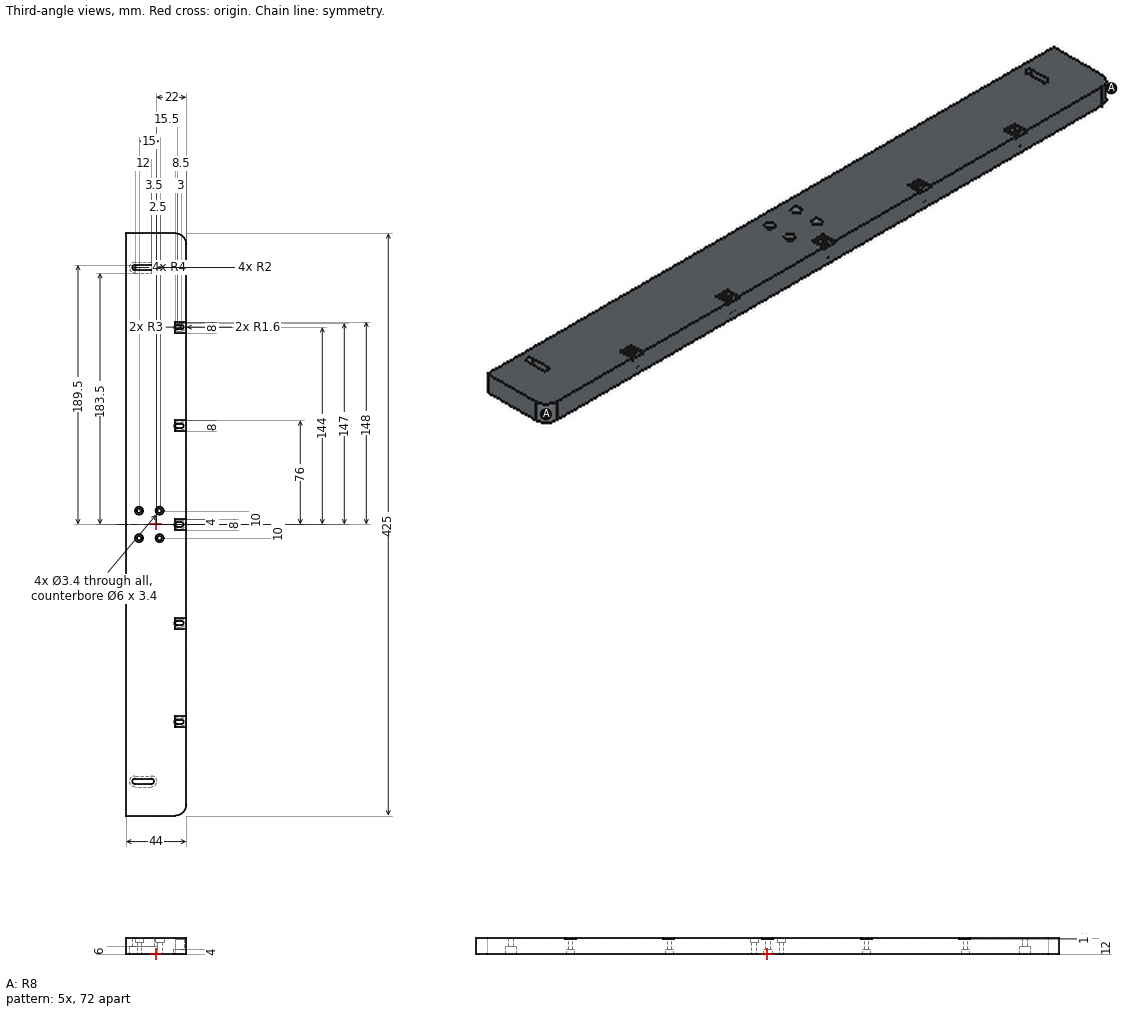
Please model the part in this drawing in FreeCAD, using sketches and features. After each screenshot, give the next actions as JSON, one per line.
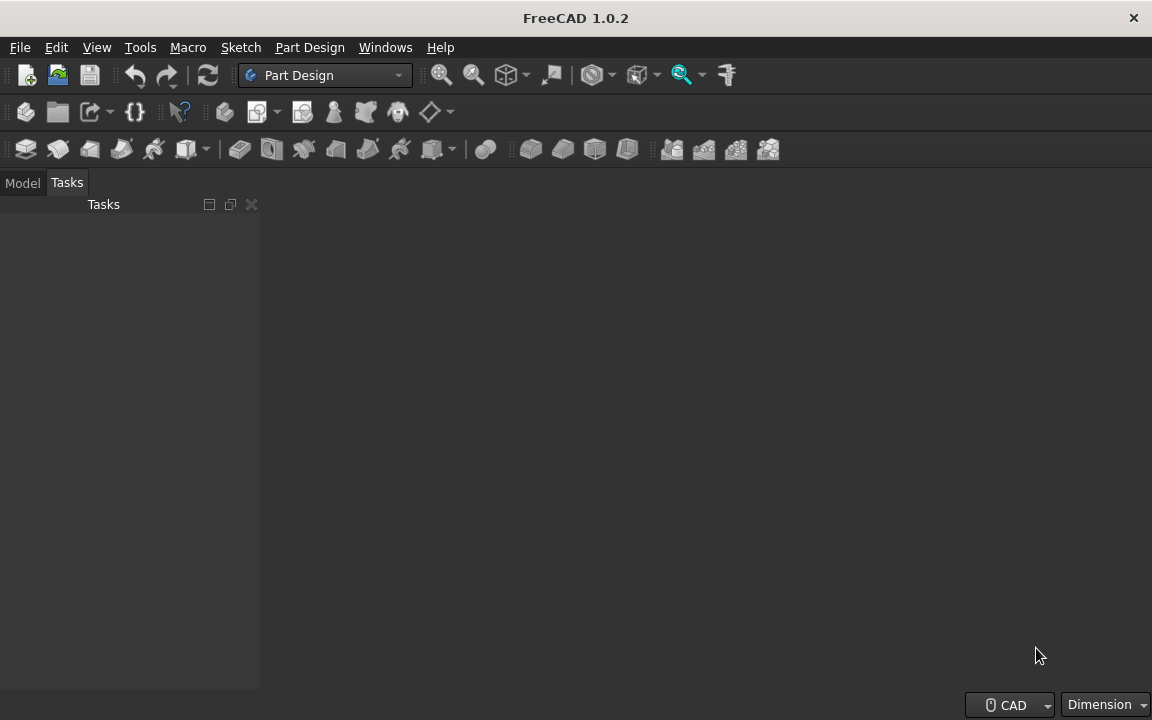
{"action": "key", "text": "ctrl+n"}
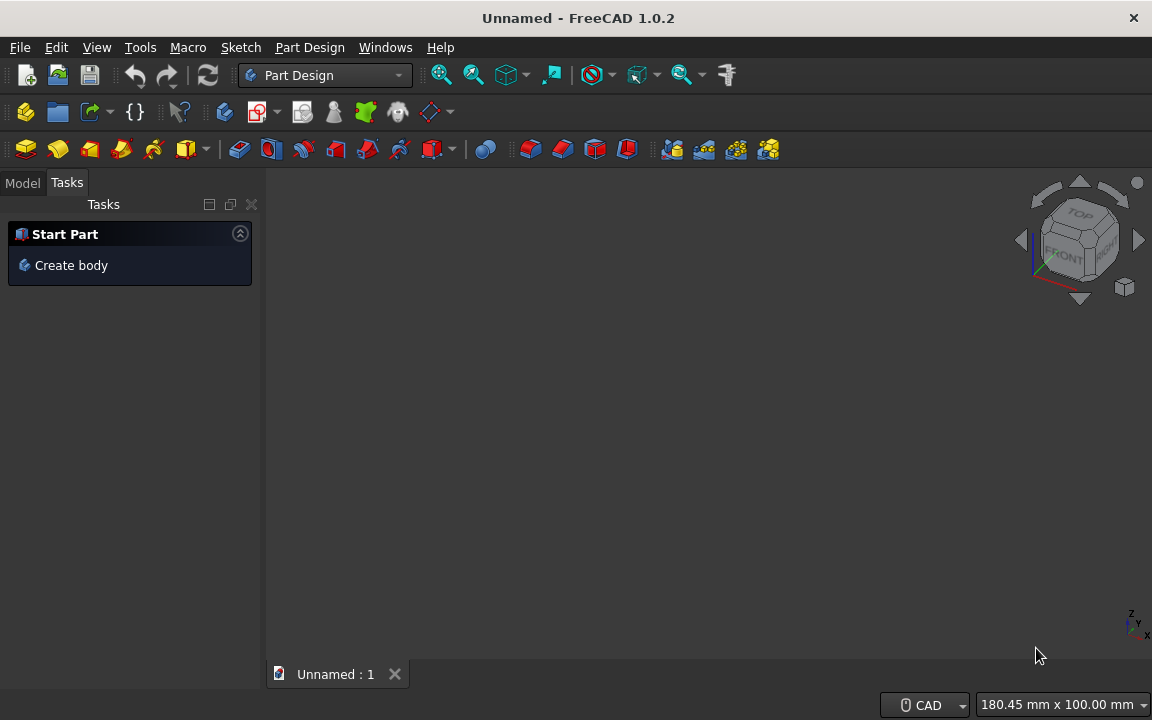
{"action": "left_click", "coordinate": [258, 112]}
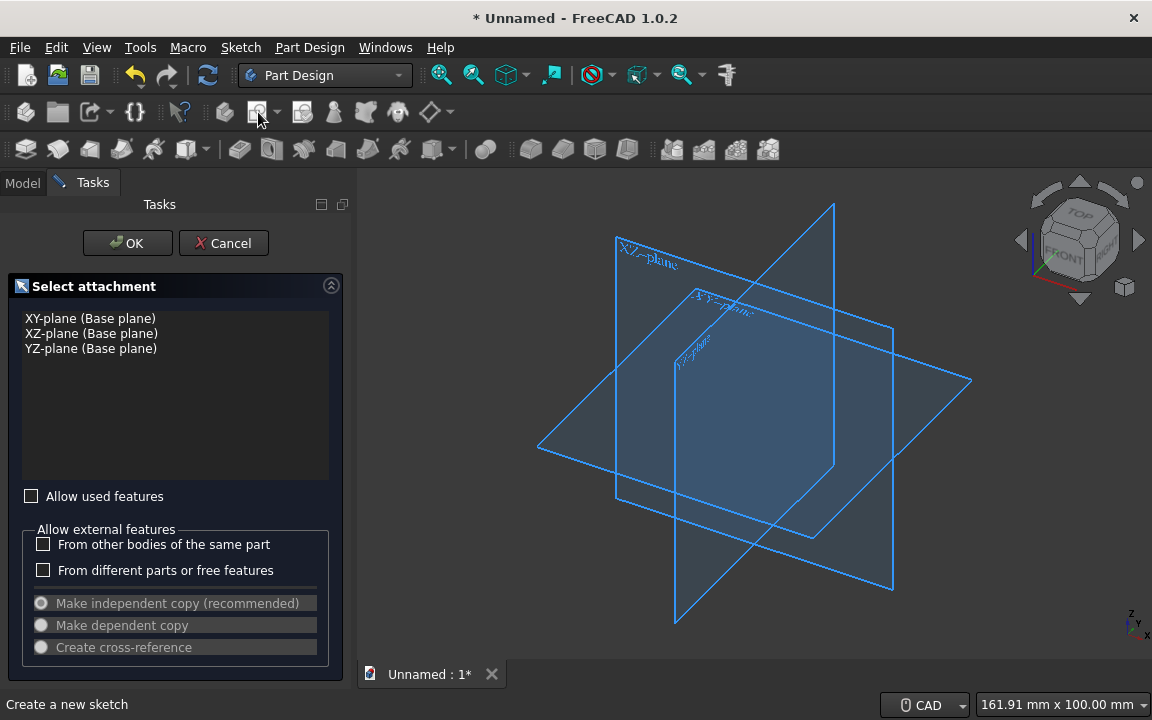
{"action": "left_click", "coordinate": [82, 318]}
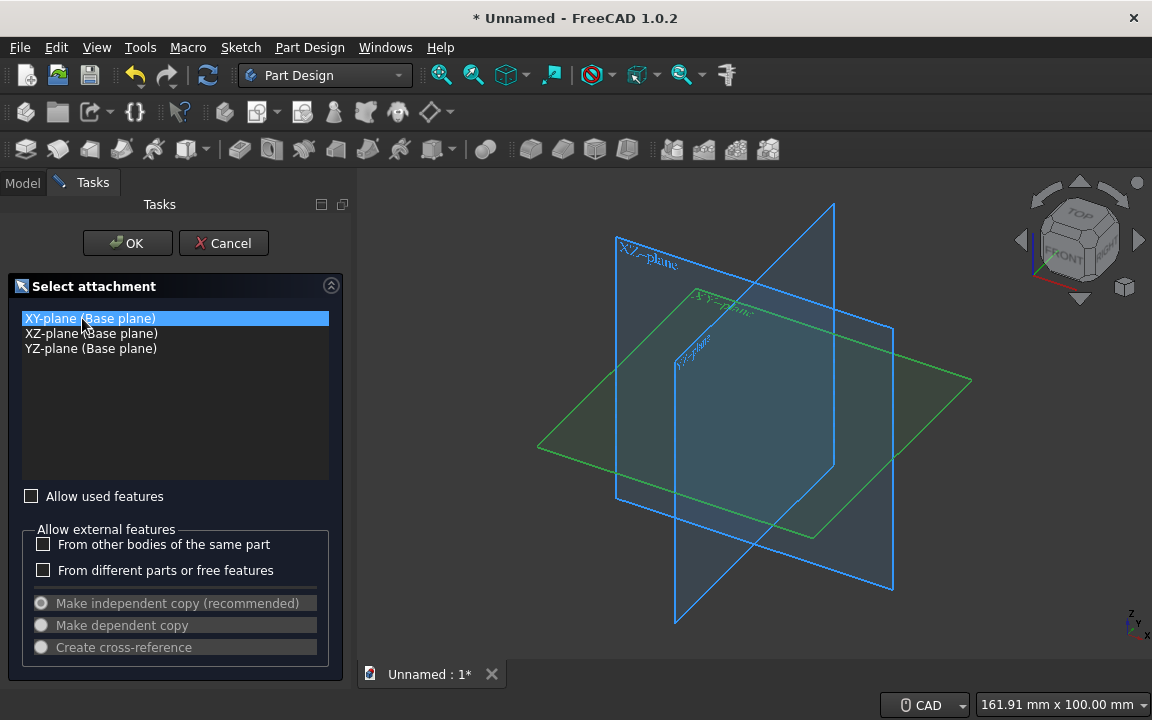
{"action": "left_click", "coordinate": [128, 243]}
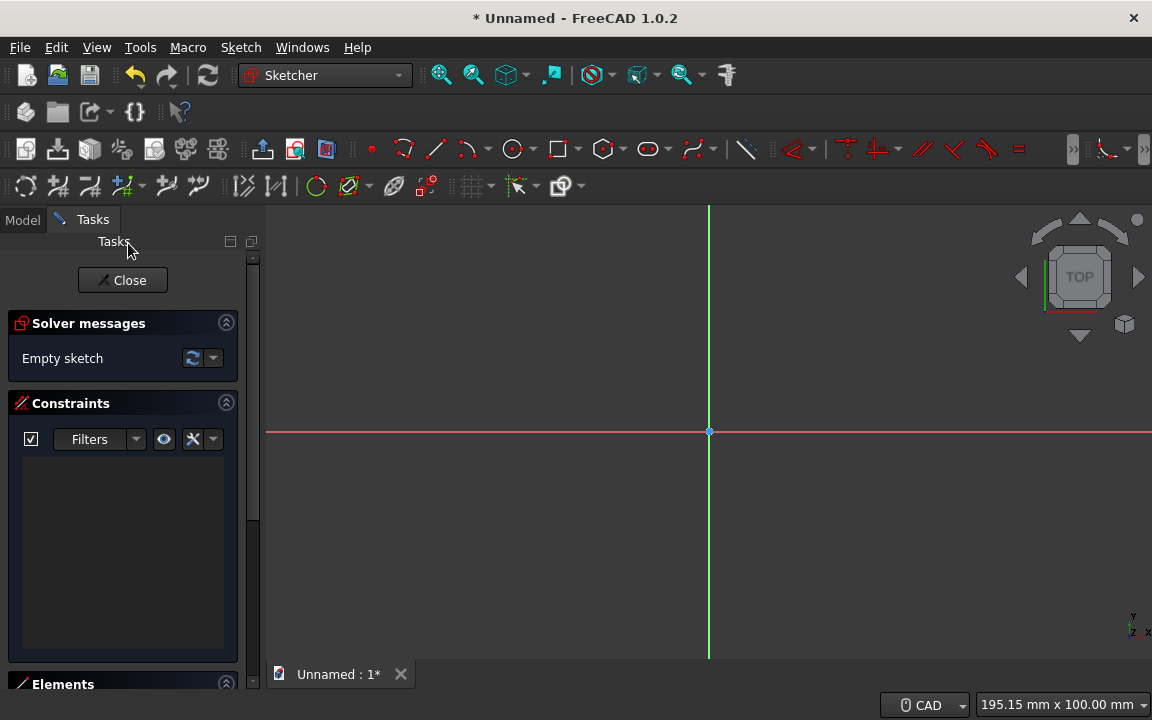
{"action": "scroll", "coordinate": [630, 432], "scroll_direction": "down", "scroll_amount": 10}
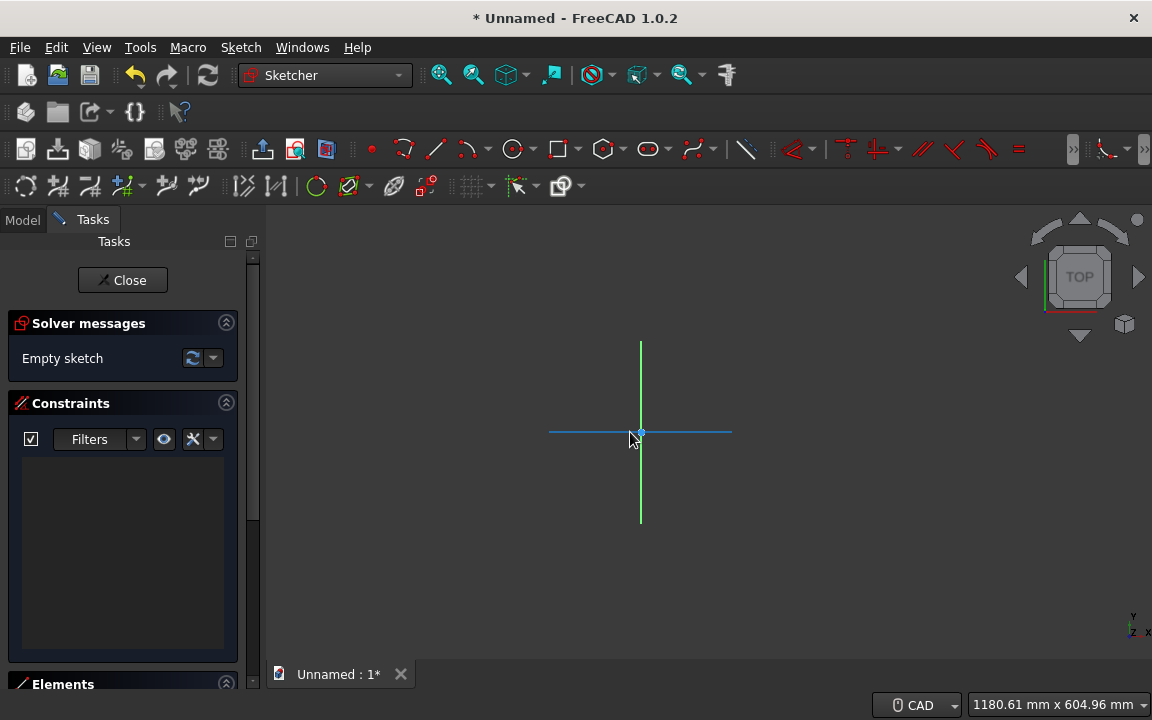
{"action": "key", "text": "g v"}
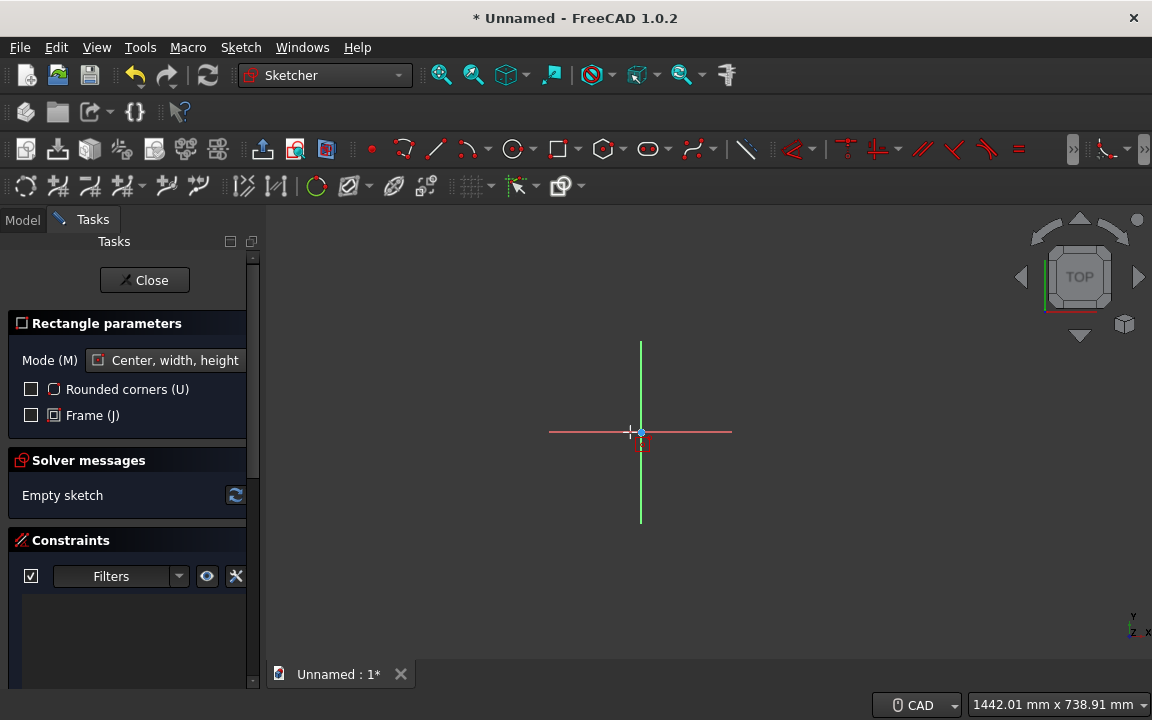
{"action": "left_click", "coordinate": [641, 432]}
{"action": "left_click", "coordinate": [655, 302]}
{"action": "key", "text": "Escape"}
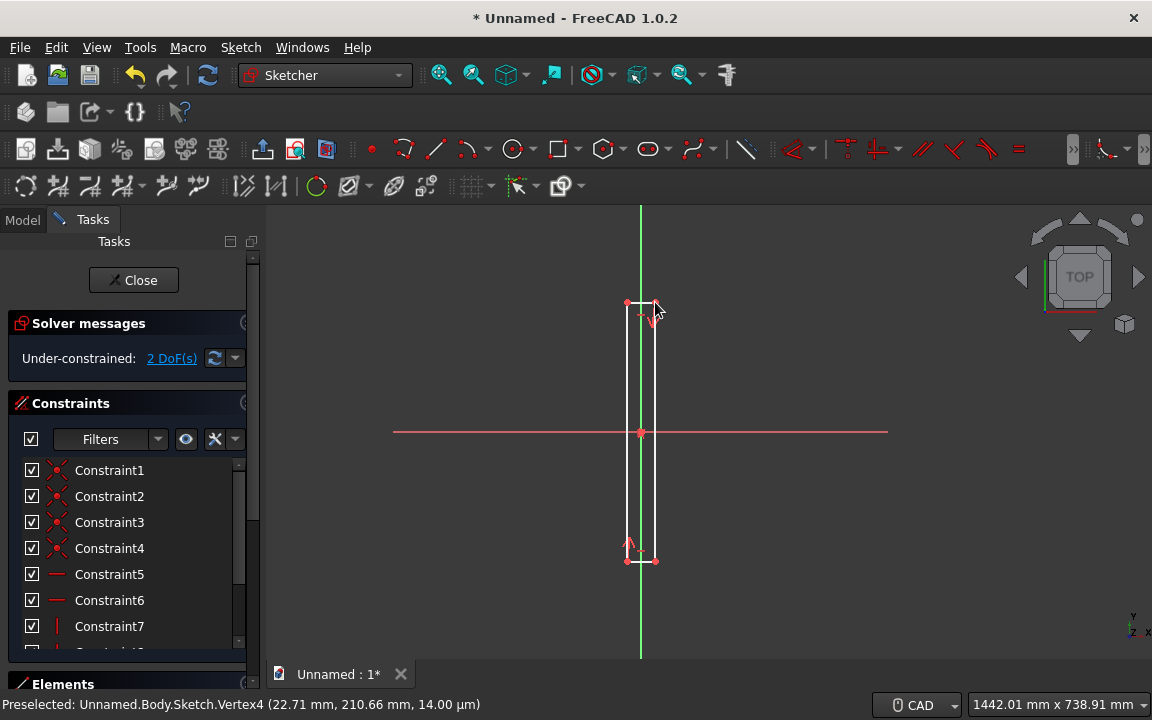
{"action": "scroll", "coordinate": [638, 562], "scroll_direction": "up", "scroll_amount": 2}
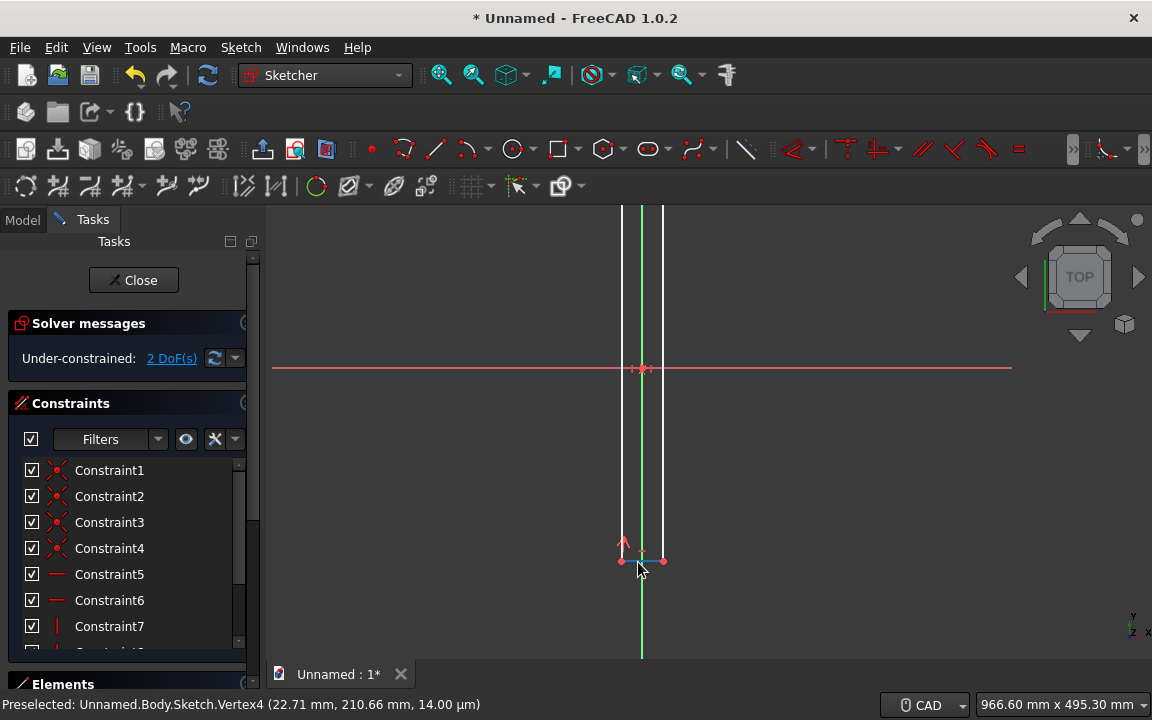
{"action": "left_click", "coordinate": [638, 561]}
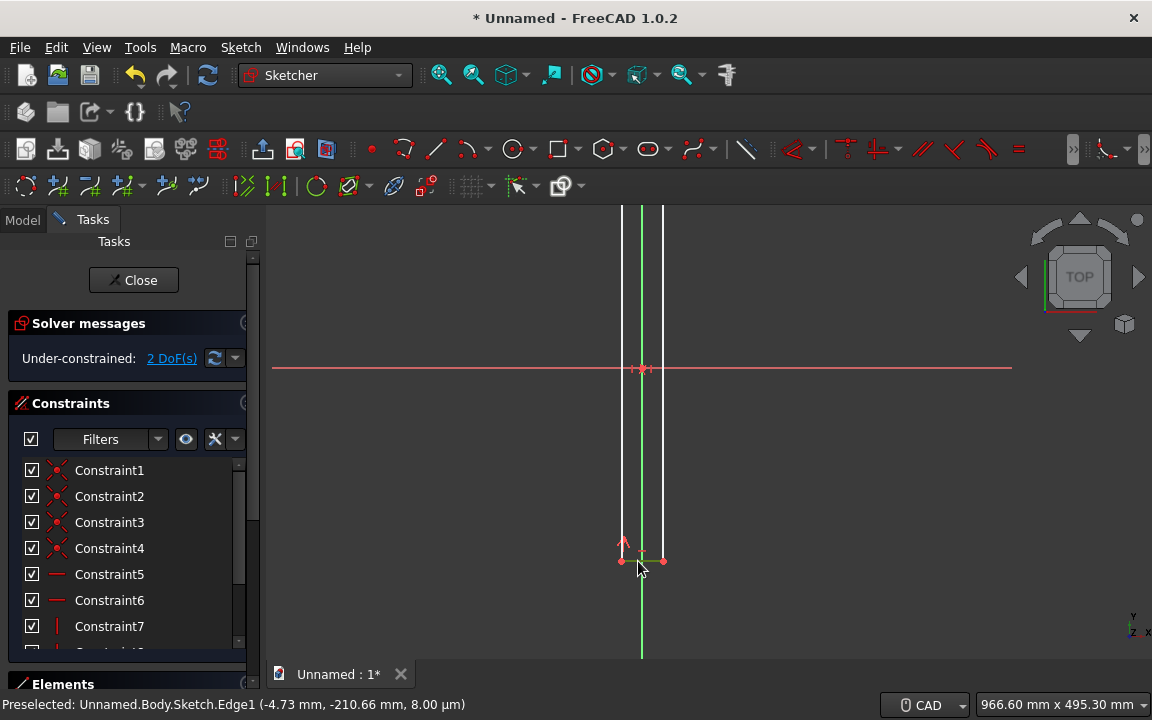
{"action": "key", "text": "l"}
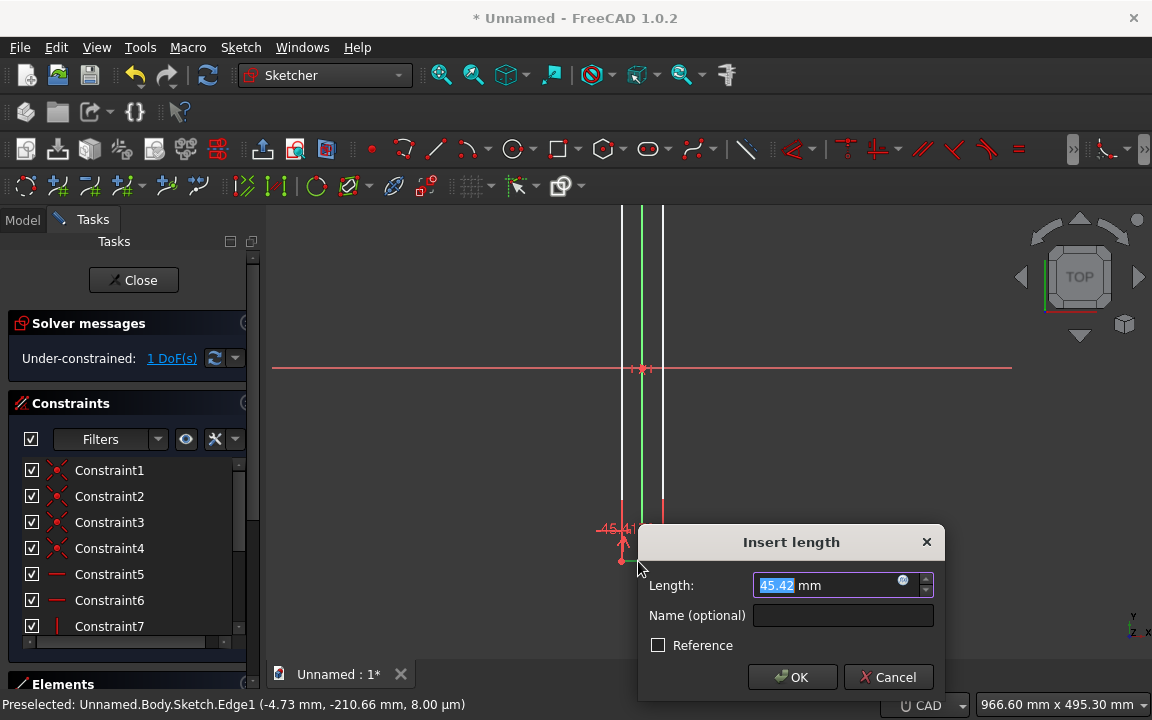
{"action": "type", "text": "44"}
{"action": "key", "text": "Return"}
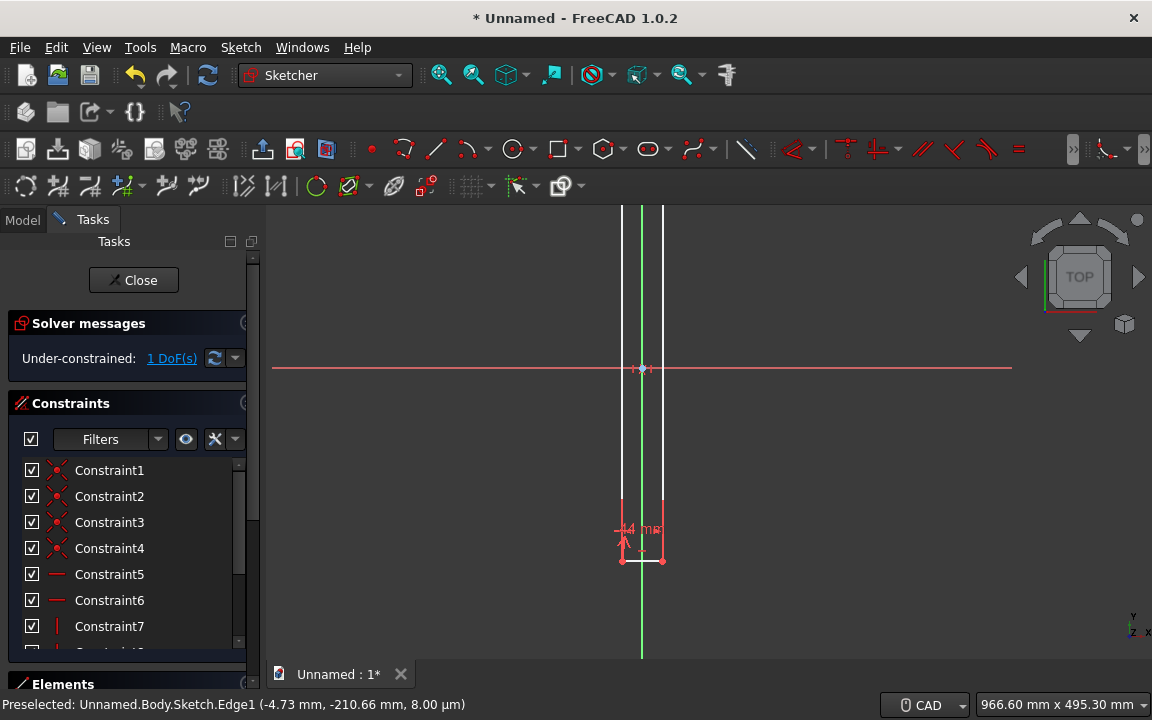
{"action": "left_click", "coordinate": [663, 446]}